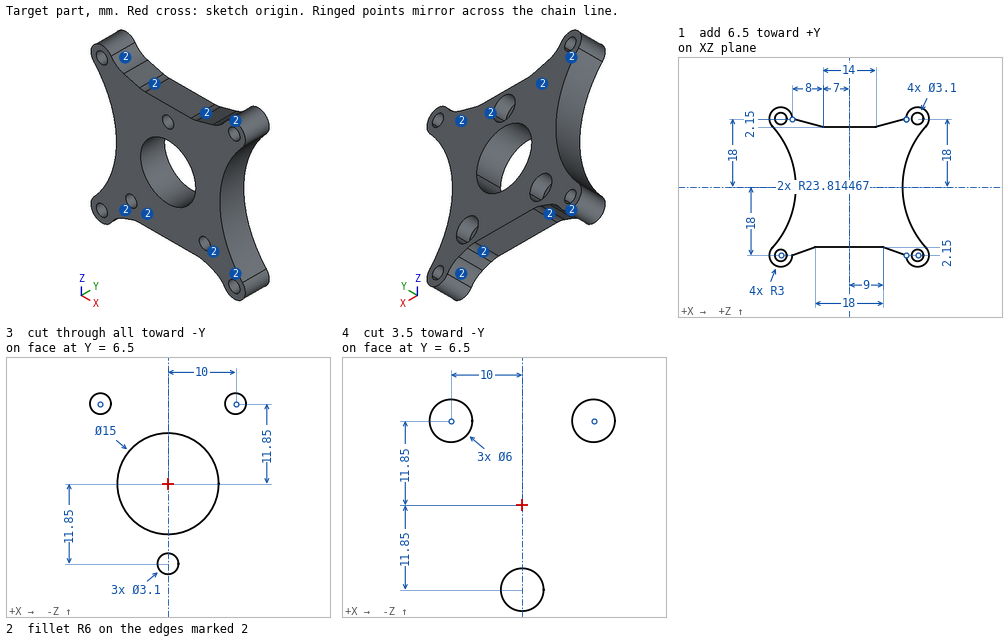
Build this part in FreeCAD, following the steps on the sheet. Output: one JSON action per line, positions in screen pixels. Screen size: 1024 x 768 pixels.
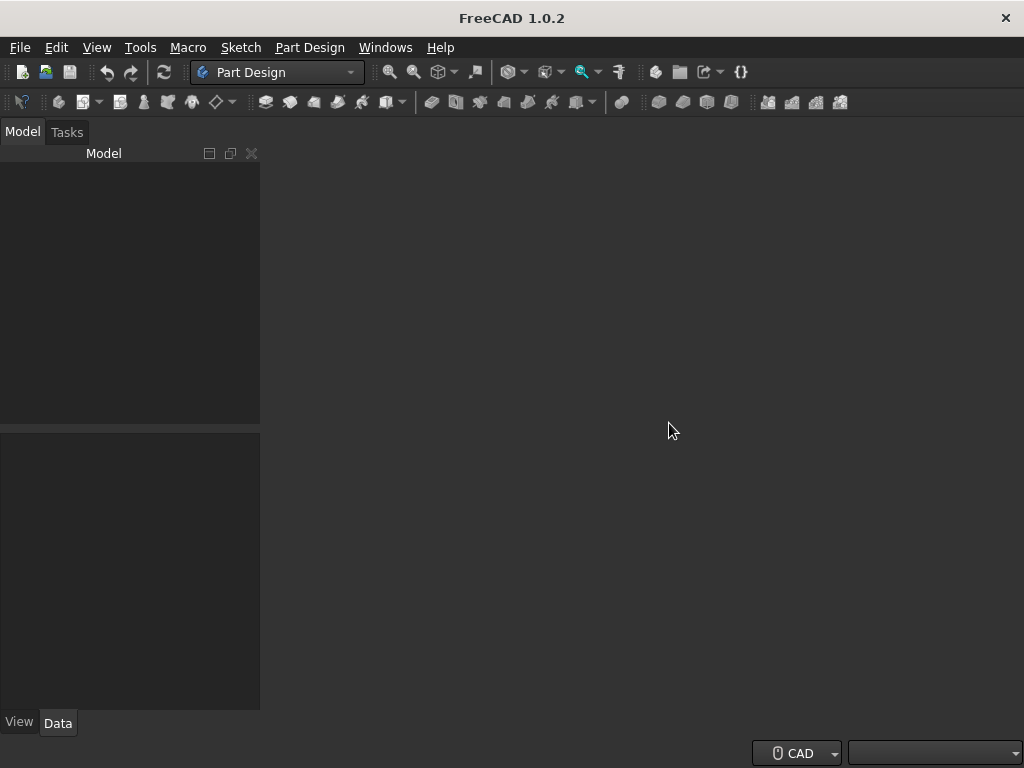
{"action": "left_click", "coordinate": [22, 72]}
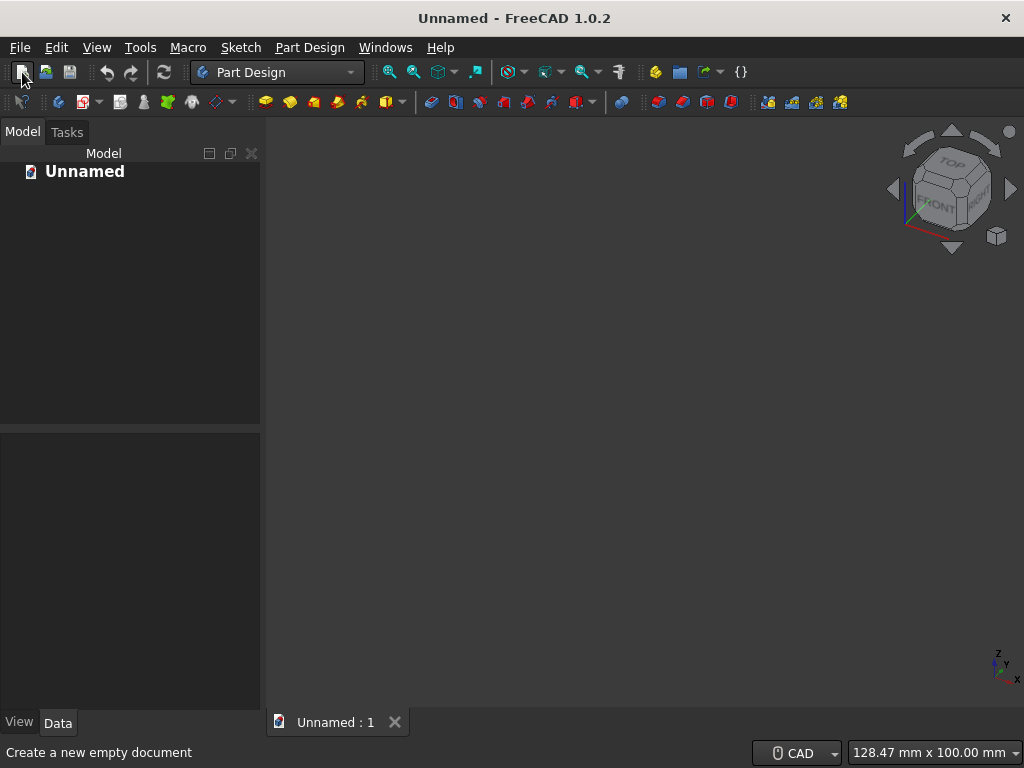
{"action": "left_click", "coordinate": [84, 102]}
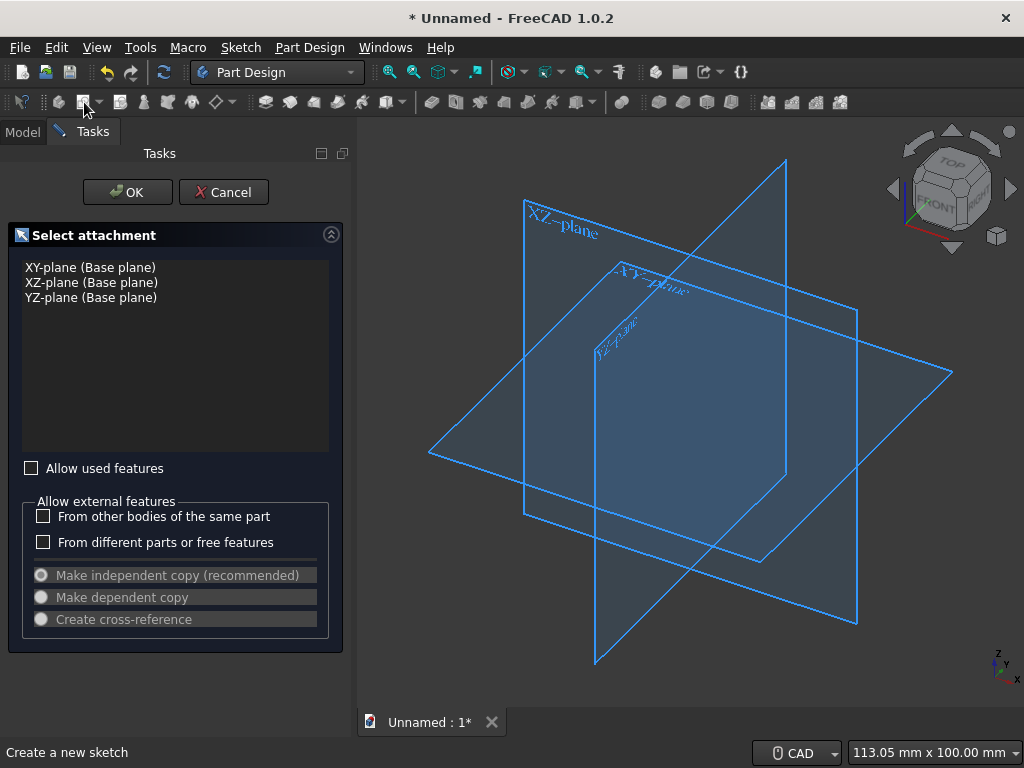
{"action": "left_click", "coordinate": [82, 282]}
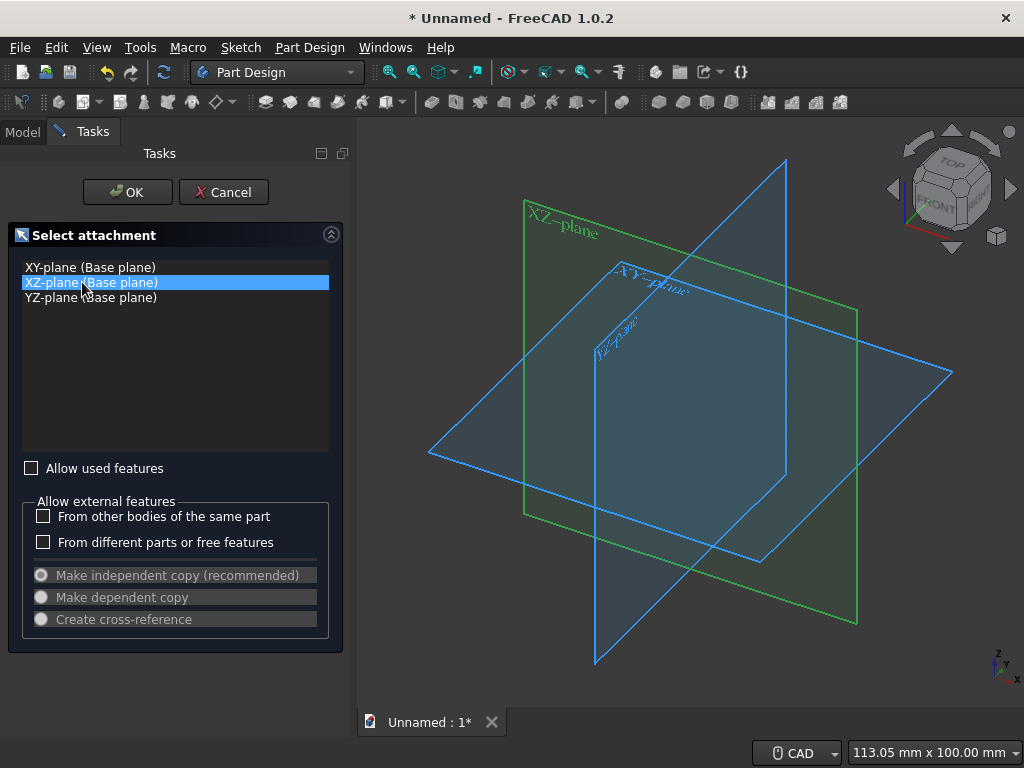
{"action": "left_click", "coordinate": [128, 192]}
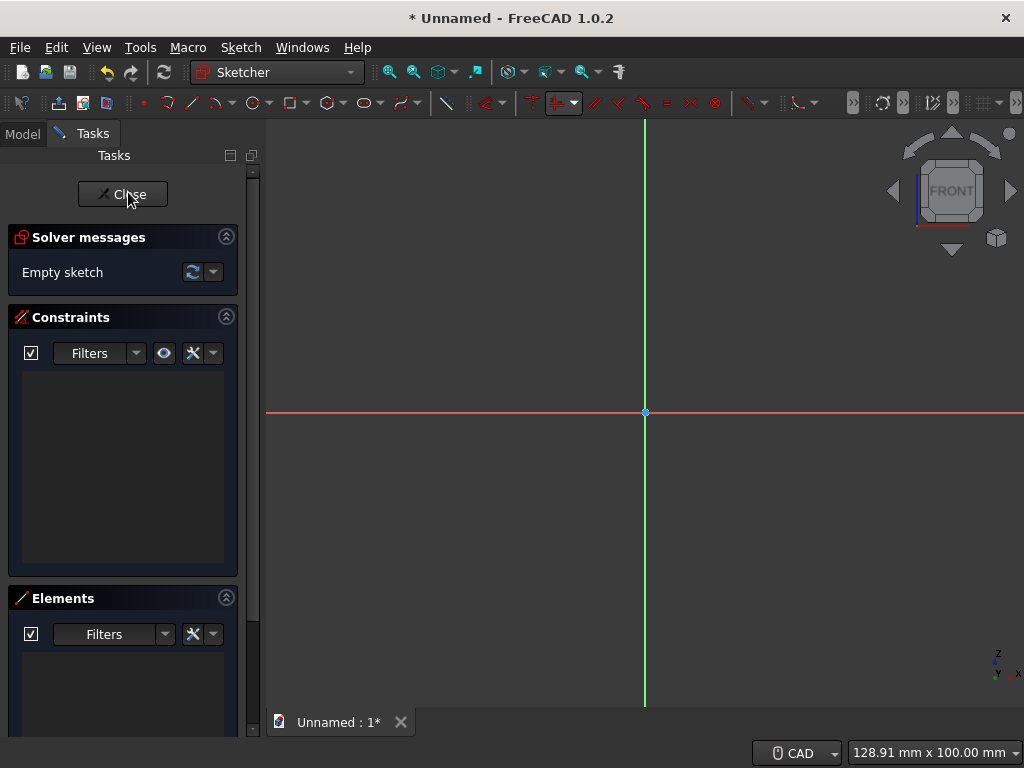
{"action": "scroll", "coordinate": [784, 413], "scroll_direction": "up", "scroll_amount": 2}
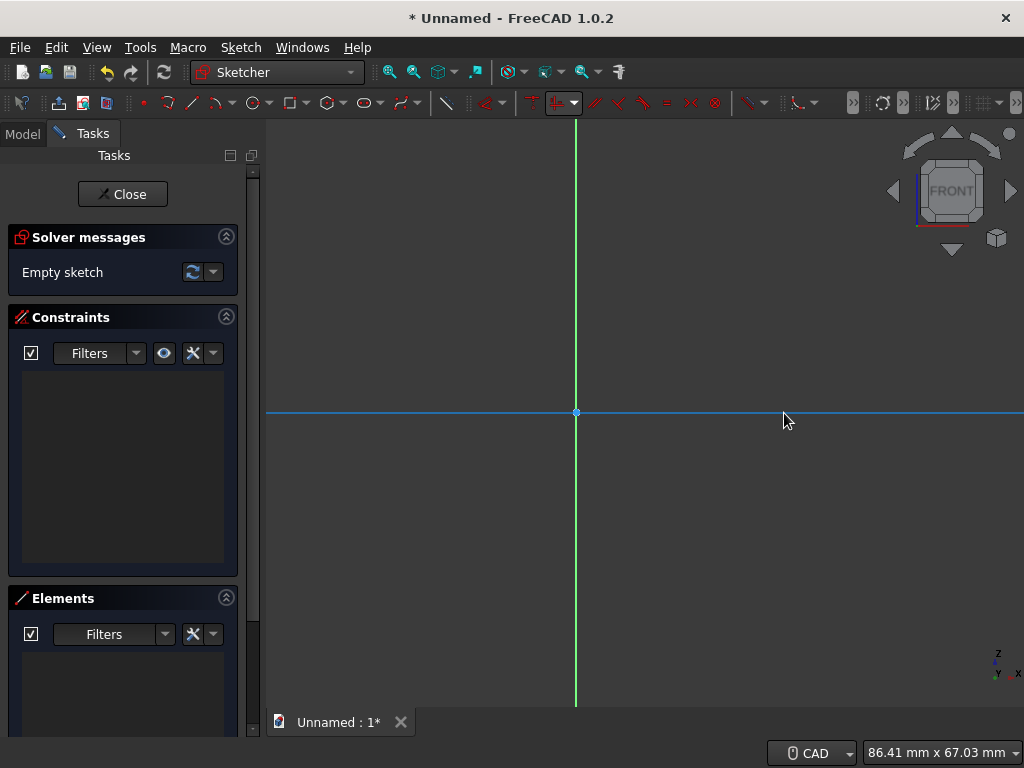
{"action": "left_click", "coordinate": [168, 104]}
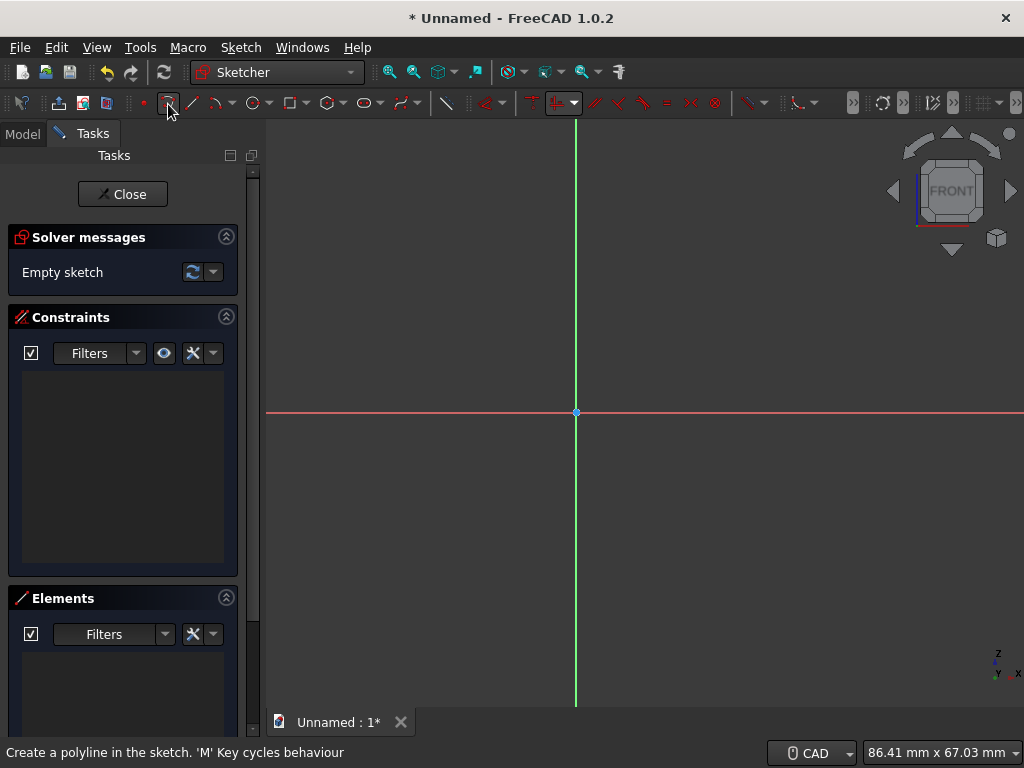
{"action": "left_click", "coordinate": [445, 255]}
{"action": "left_click", "coordinate": [515, 274]}
{"action": "left_click", "coordinate": [638, 274]}
{"action": "left_click", "coordinate": [708, 255]}
{"action": "right_click", "coordinate": [708, 255]}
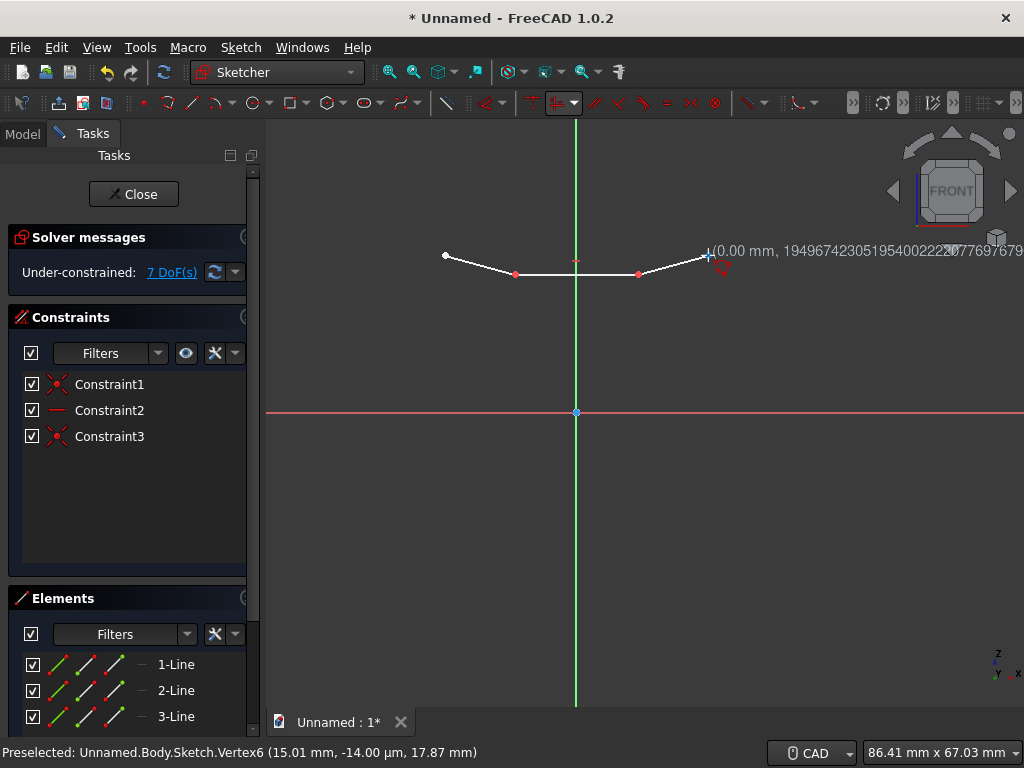
{"action": "left_click", "coordinate": [708, 571]}
{"action": "left_click", "coordinate": [655, 552]}
{"action": "left_click", "coordinate": [497, 552]}
{"action": "left_click", "coordinate": [445, 571]}
{"action": "right_click", "coordinate": [445, 571]}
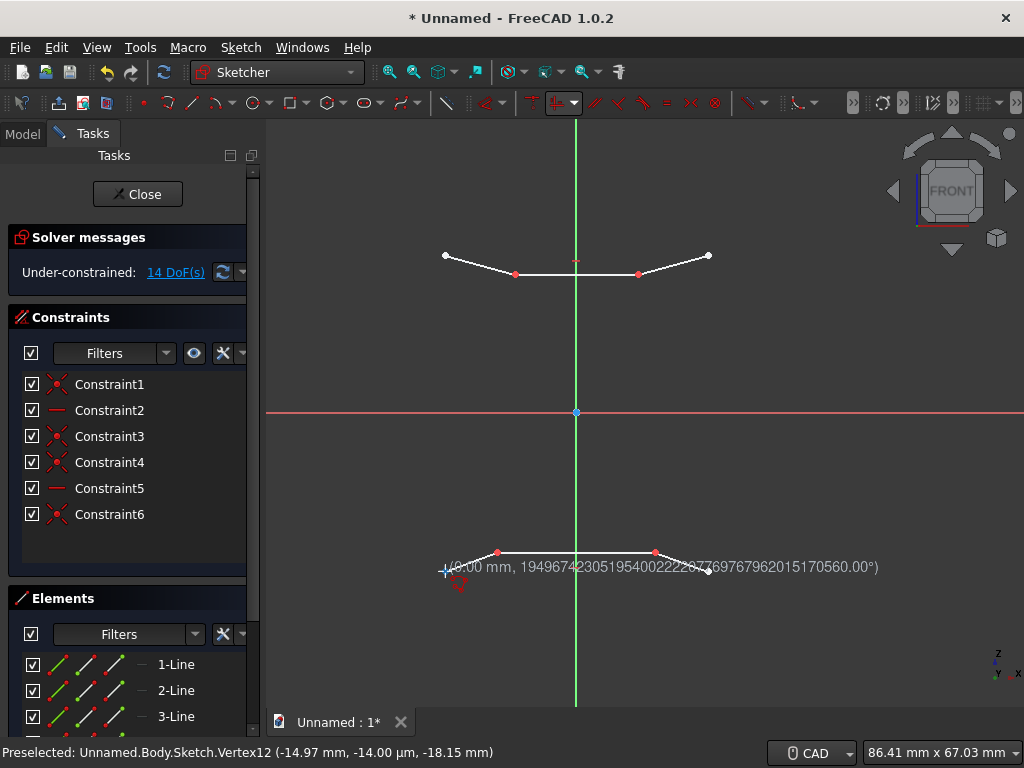
{"action": "left_click", "coordinate": [234, 104]}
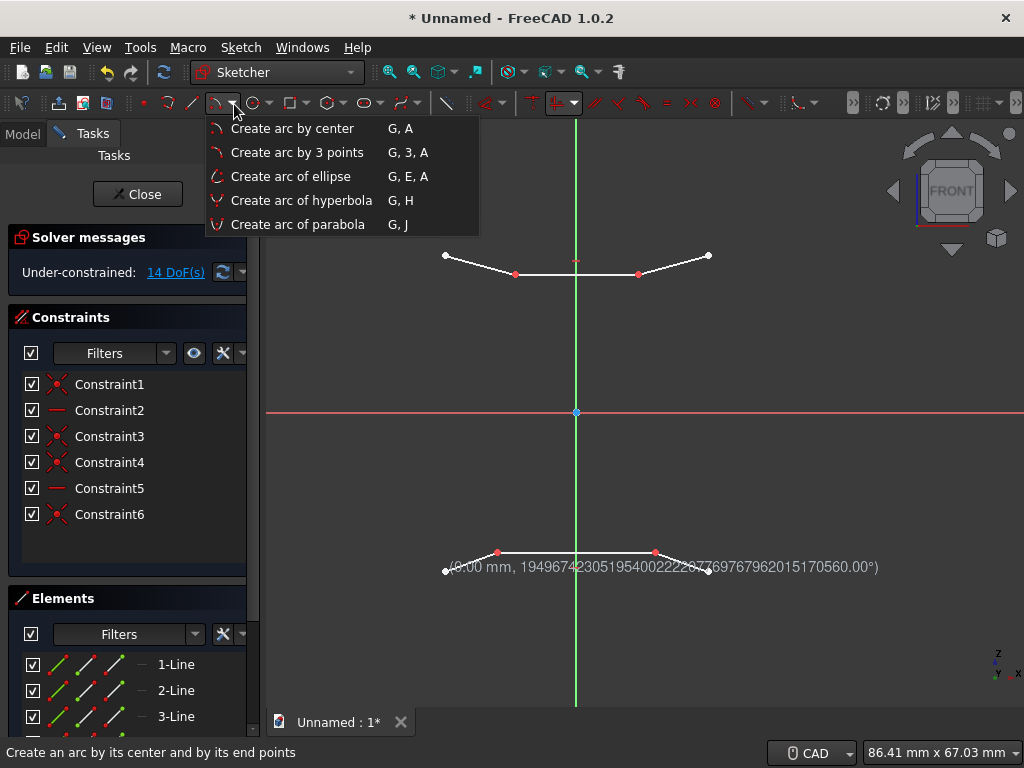
{"action": "left_click", "coordinate": [342, 152]}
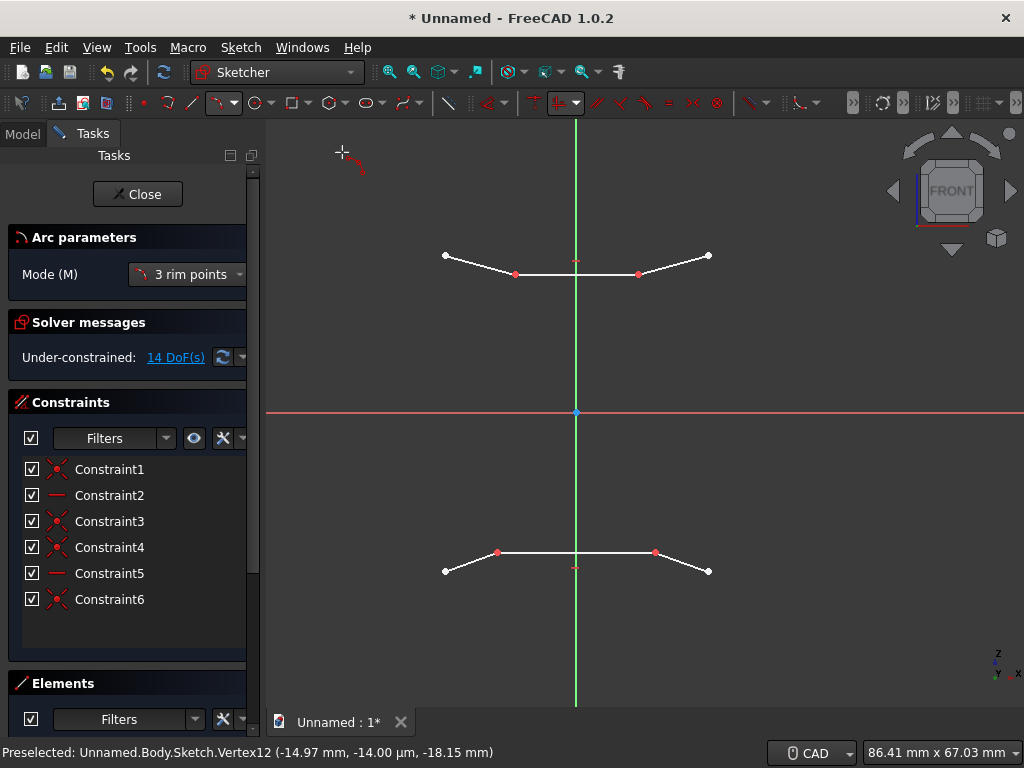
{"action": "left_click", "coordinate": [708, 256]}
{"action": "left_click", "coordinate": [754, 273]}
{"action": "left_click", "coordinate": [744, 230]}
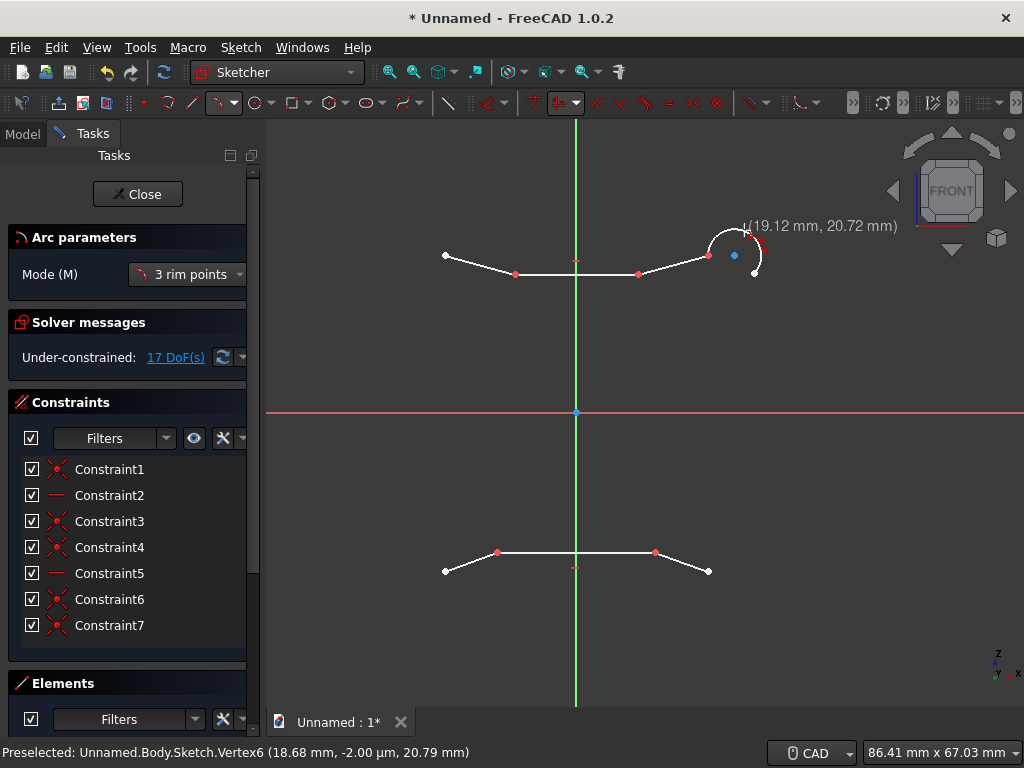
{"action": "left_click", "coordinate": [754, 274]}
{"action": "left_click", "coordinate": [754, 553]}
{"action": "left_click", "coordinate": [702, 382]}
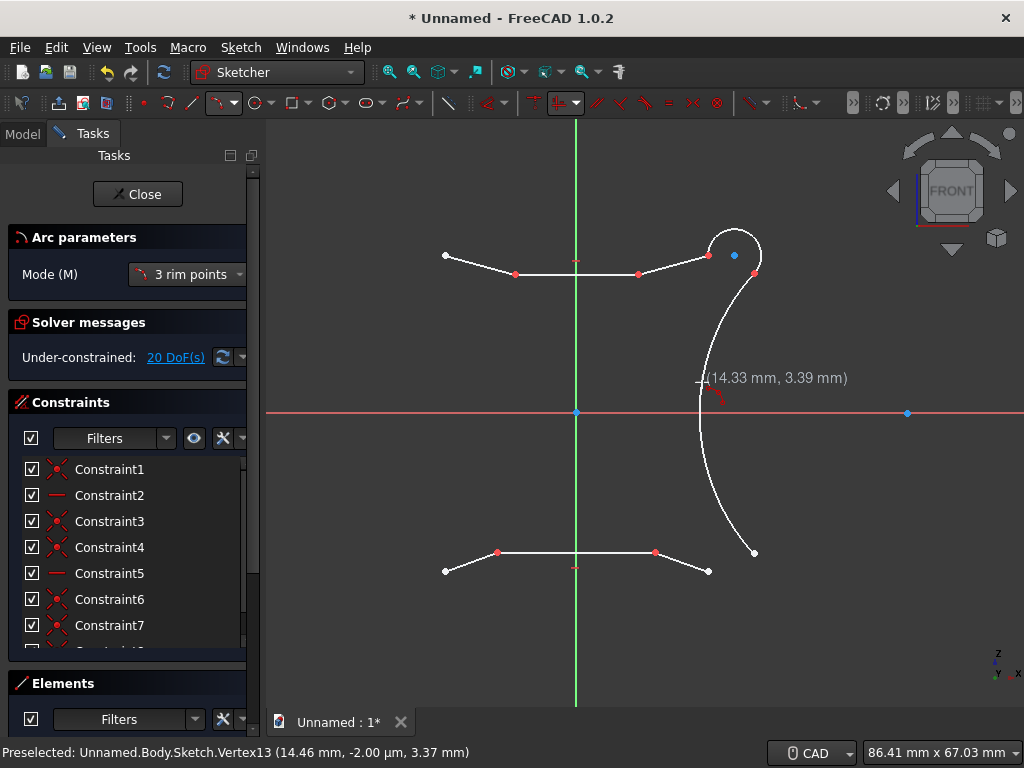
{"action": "left_click", "coordinate": [754, 554]}
{"action": "left_click", "coordinate": [708, 572]}
{"action": "left_click", "coordinate": [744, 595]}